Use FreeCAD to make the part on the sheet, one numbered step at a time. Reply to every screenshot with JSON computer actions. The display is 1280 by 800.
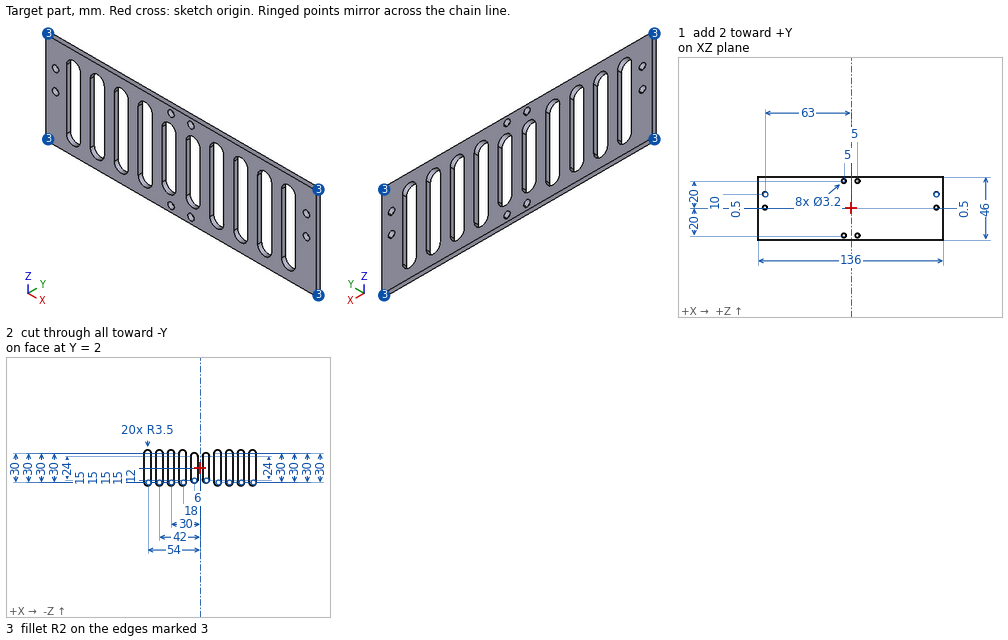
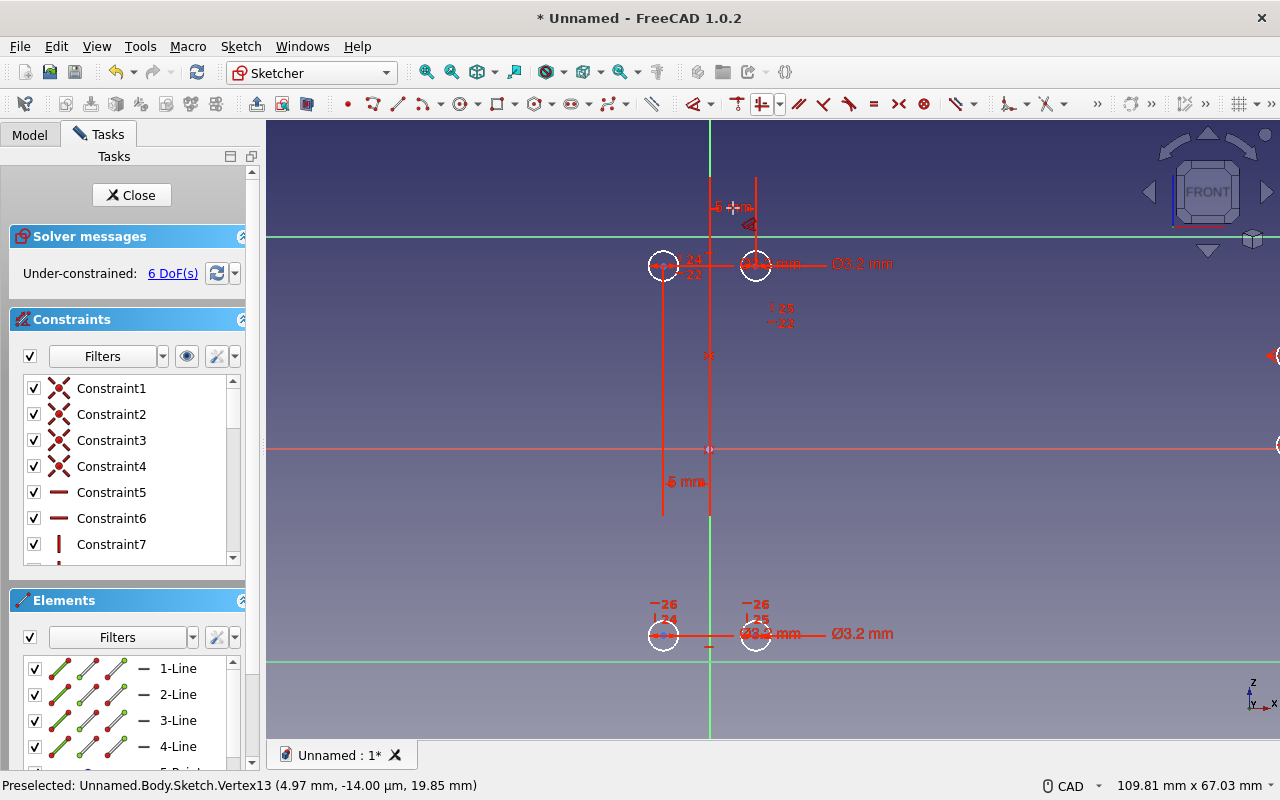
{"action": "left_click", "coordinate": [663, 266]}
{"action": "left_click", "coordinate": [629, 358]}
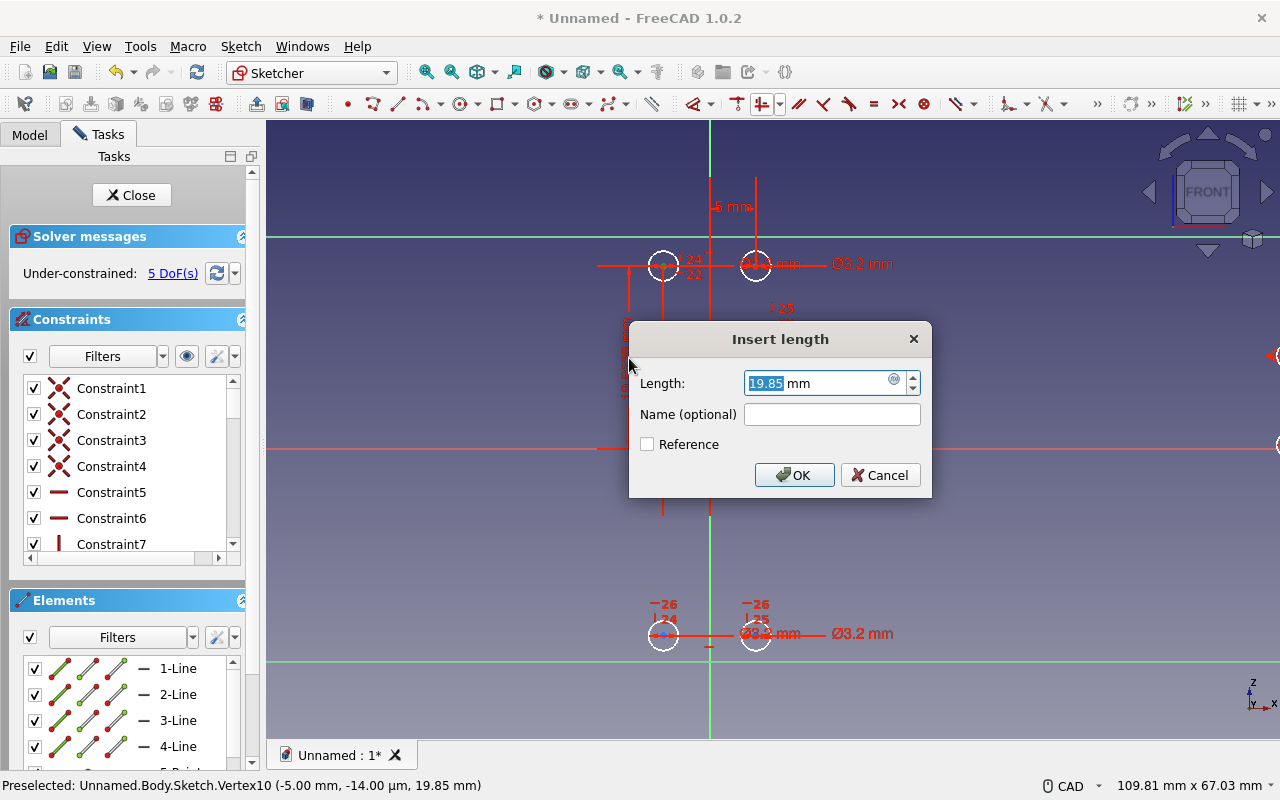
{"action": "type", "text": "20"}
{"action": "key", "text": "Return"}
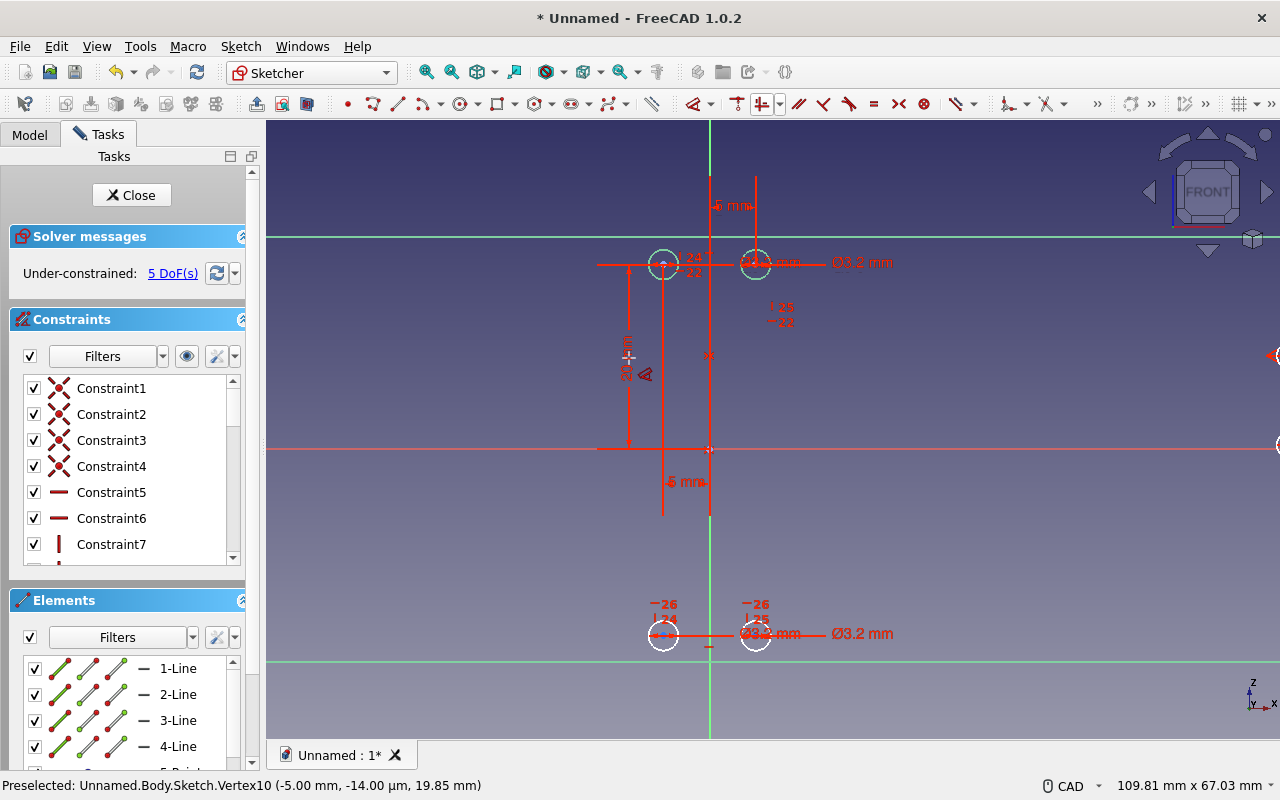
{"action": "scroll", "coordinate": [700, 413], "scroll_direction": "down", "scroll_amount": 4}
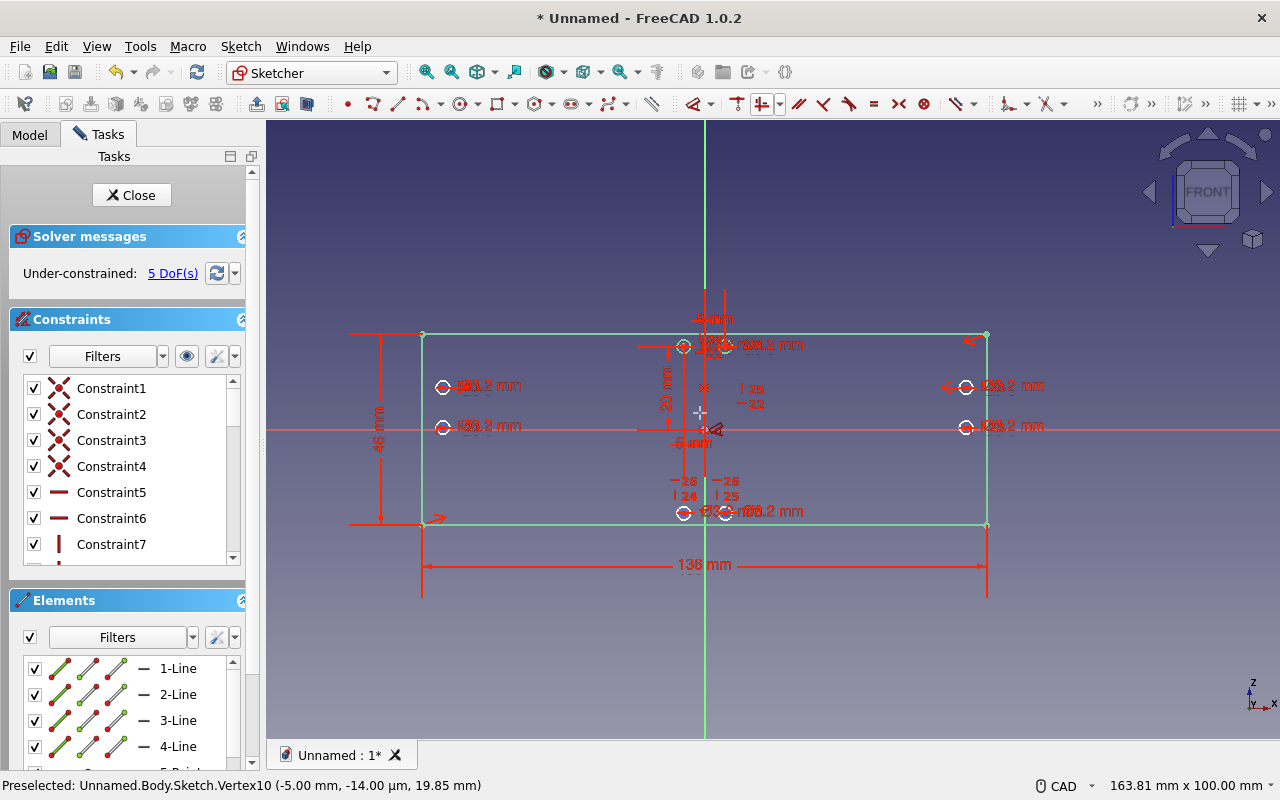
{"action": "left_click", "coordinate": [443, 388]}
{"action": "left_click", "coordinate": [574, 354]}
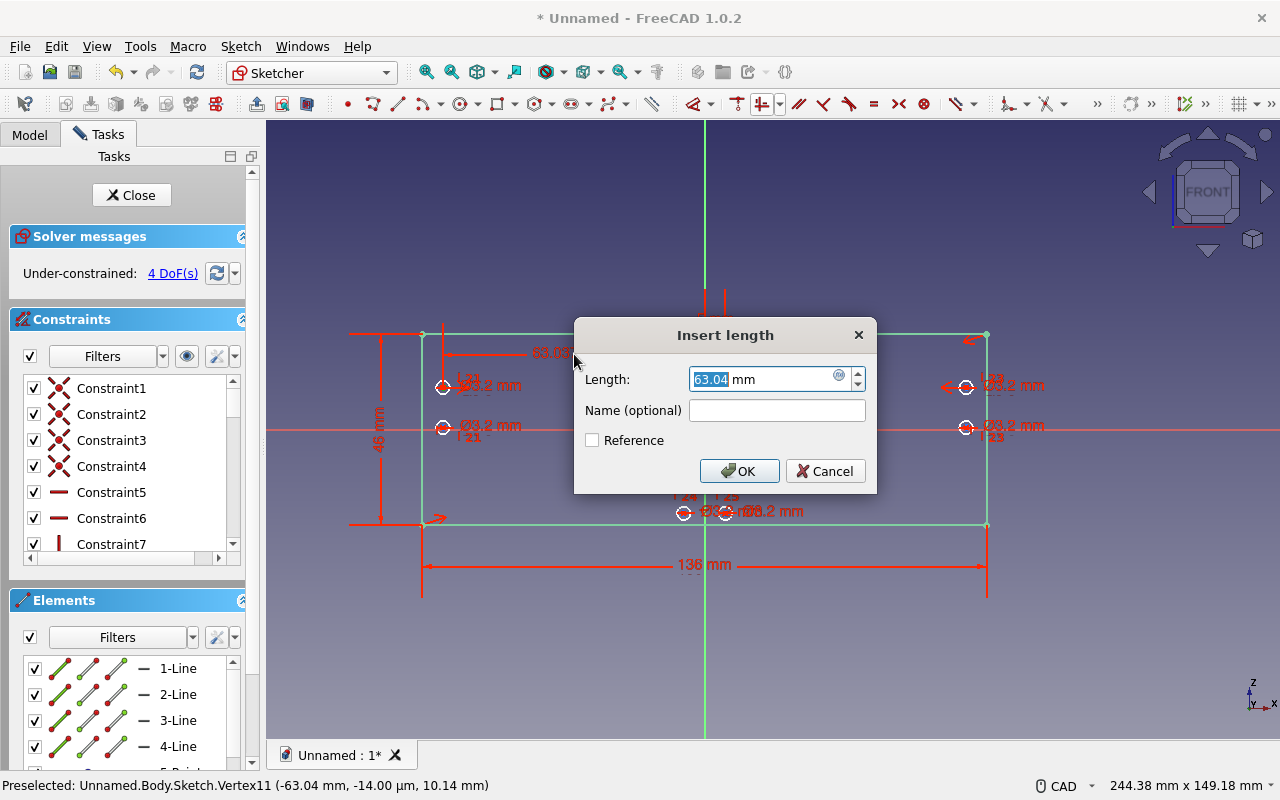
{"action": "type", "text": "63"}
{"action": "key", "text": "Return"}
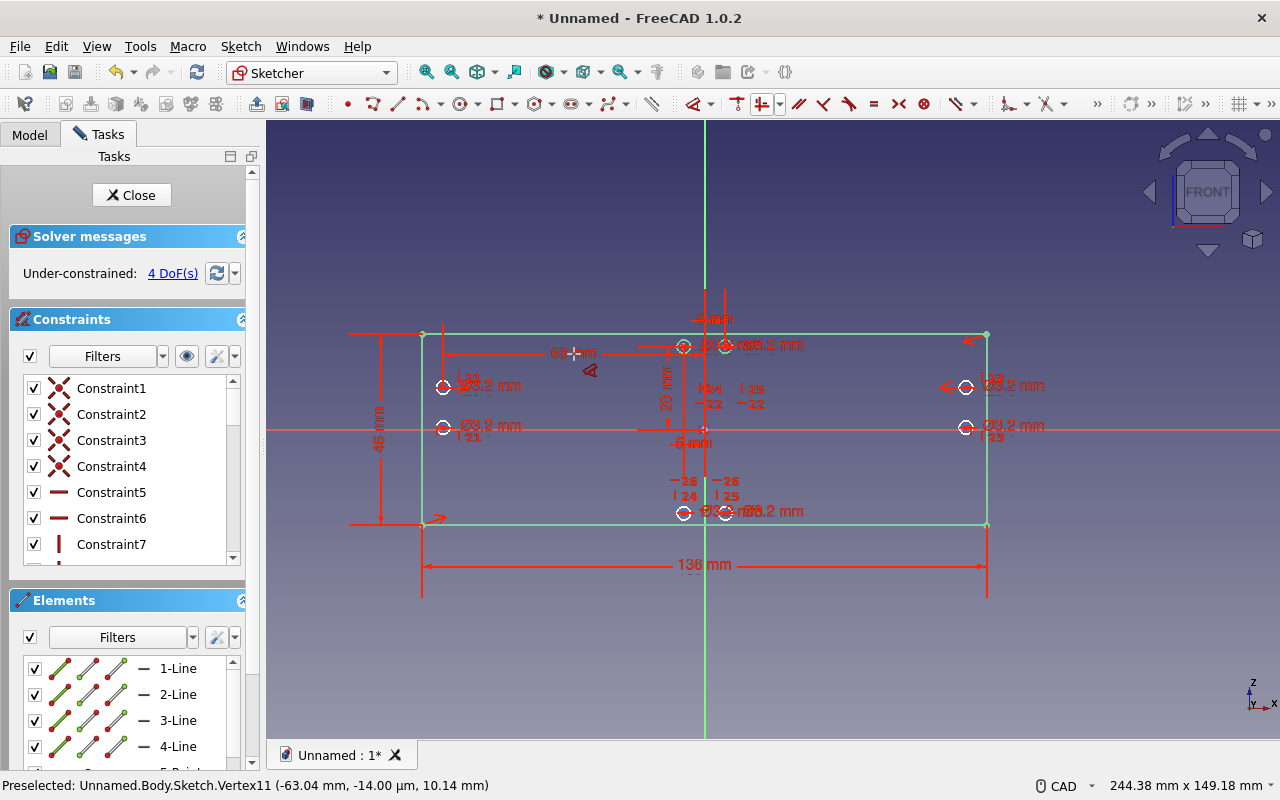
{"action": "left_click", "coordinate": [684, 513]}
{"action": "left_click", "coordinate": [650, 471]}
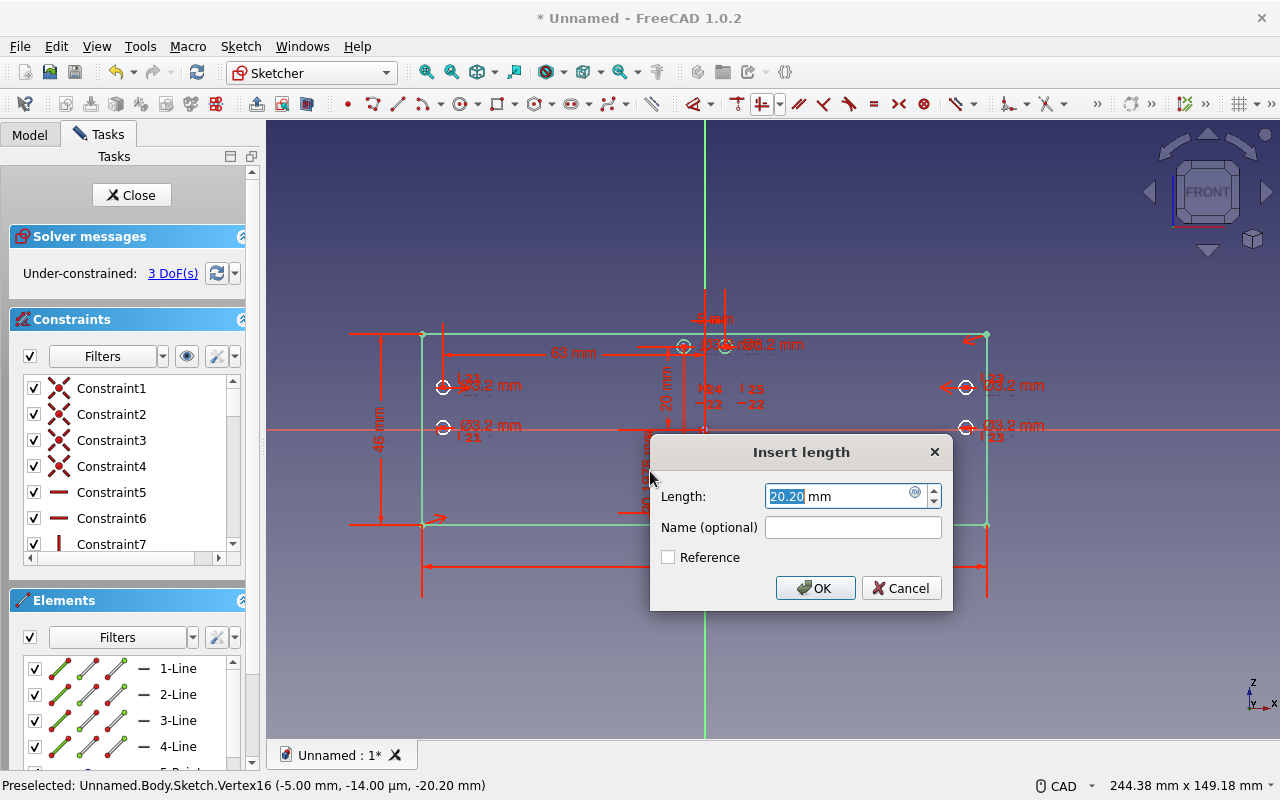
{"action": "type", "text": "20"}
{"action": "key", "text": "Return"}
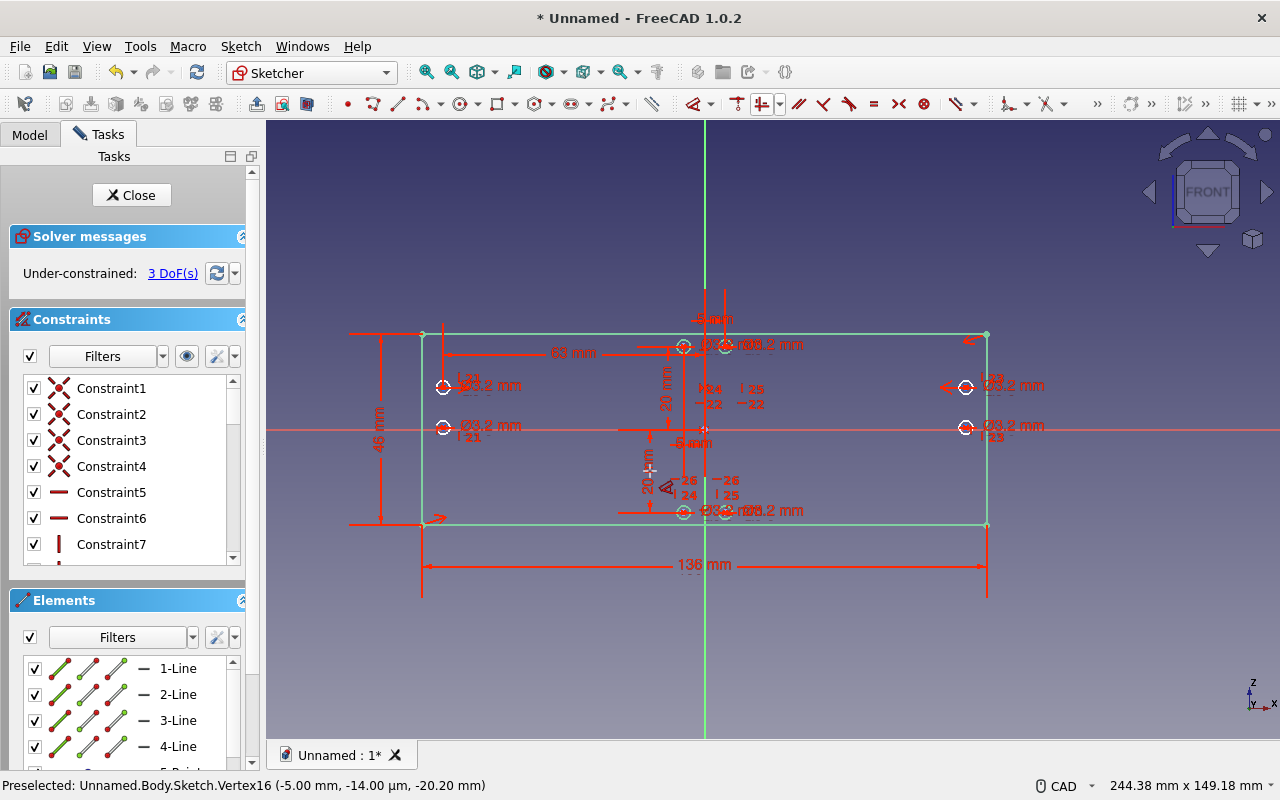
{"action": "scroll", "coordinate": [443, 428], "scroll_direction": "up", "scroll_amount": 15}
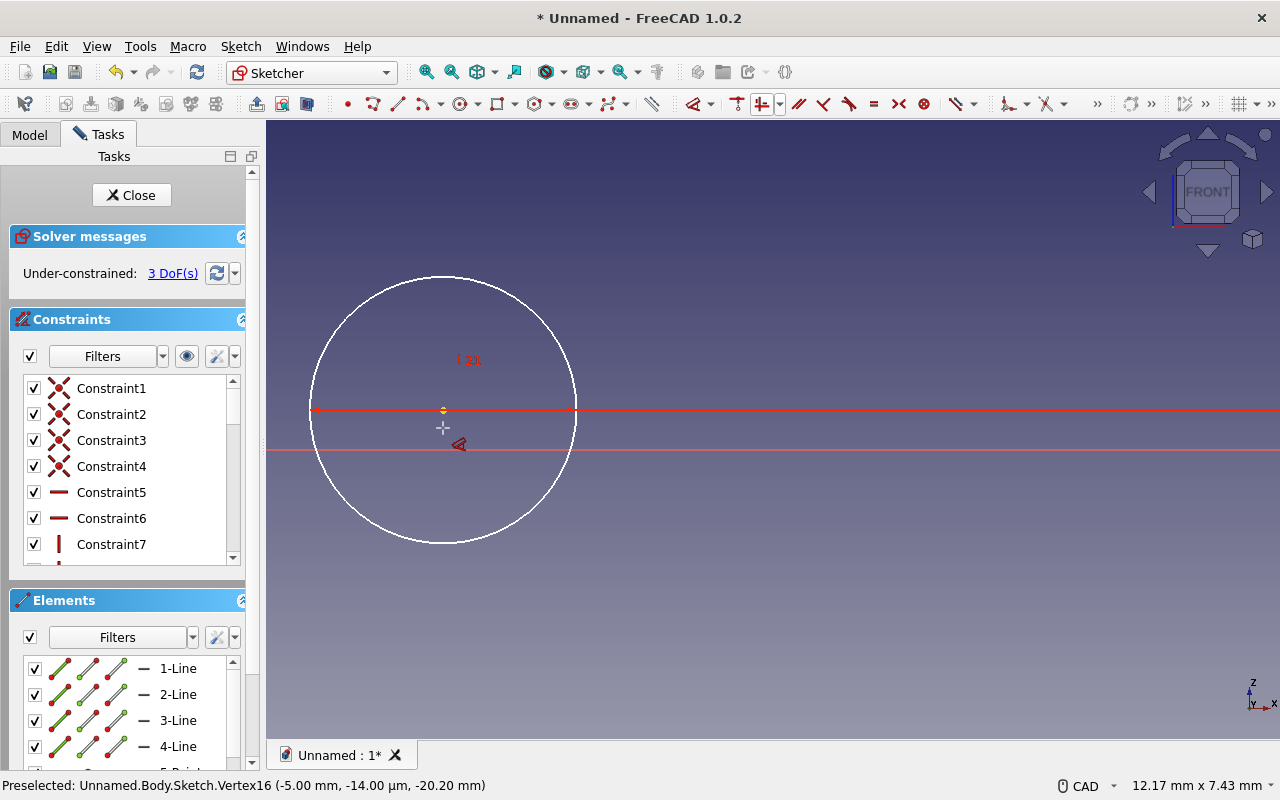
{"action": "left_click", "coordinate": [443, 410]}
{"action": "left_click", "coordinate": [409, 430]}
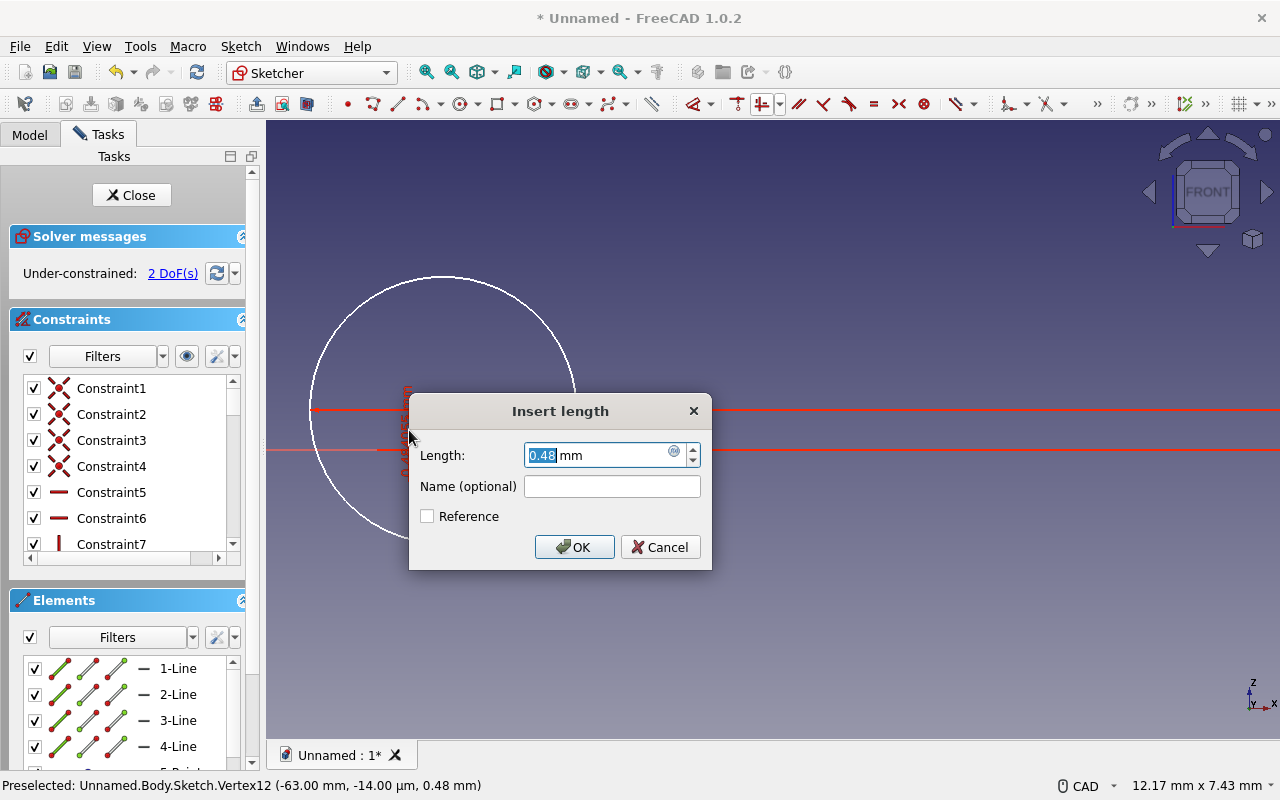
{"action": "type", "text": "0.5"}
{"action": "key", "text": "Return"}